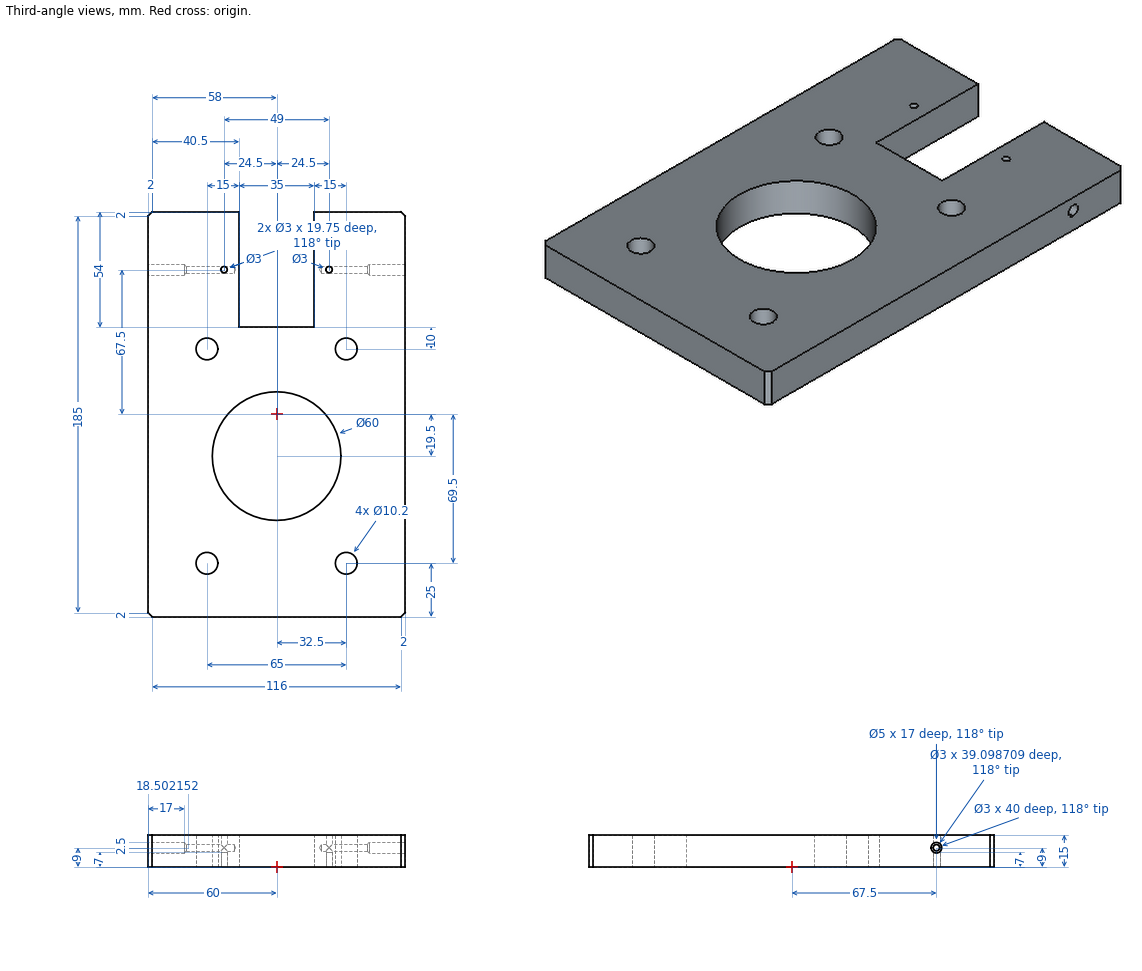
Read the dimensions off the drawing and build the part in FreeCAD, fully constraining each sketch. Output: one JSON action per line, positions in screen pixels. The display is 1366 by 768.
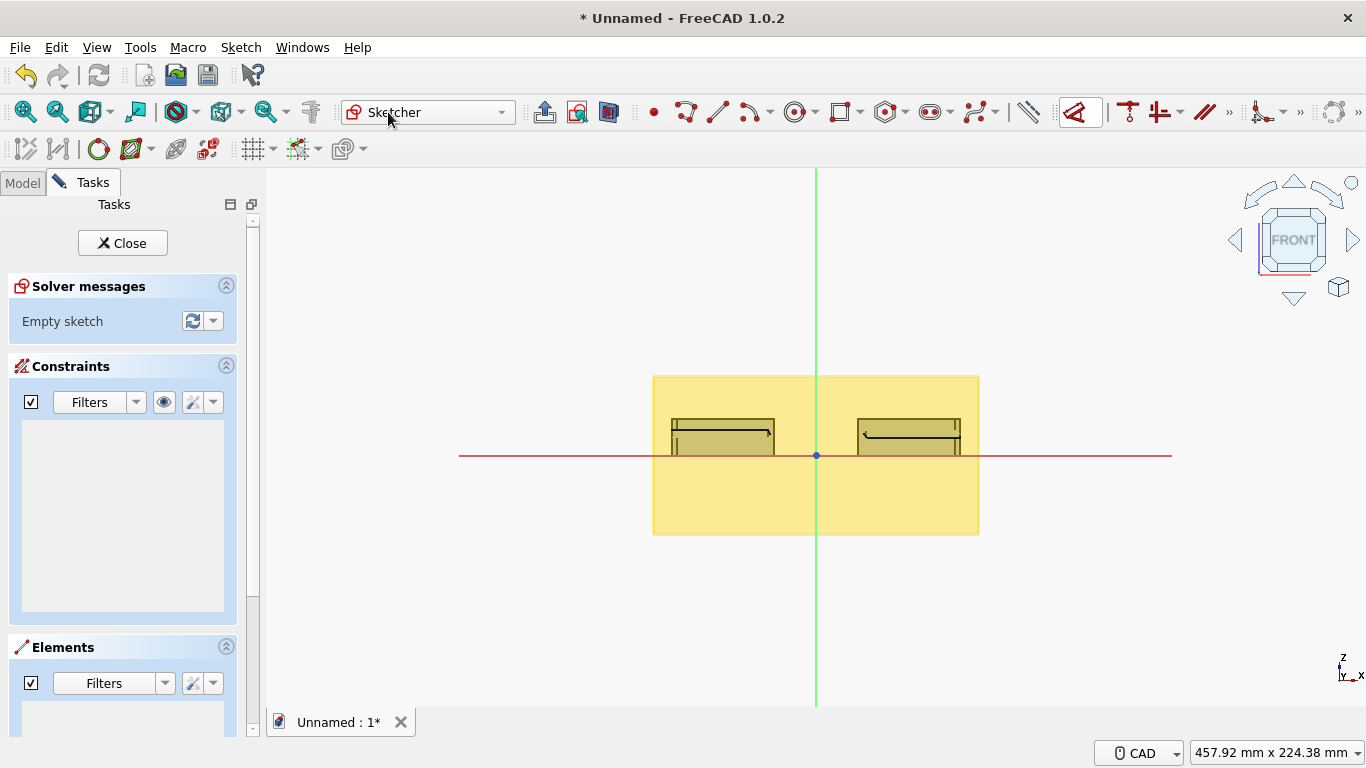
{"action": "scroll", "coordinate": [743, 443], "scroll_direction": "up", "scroll_amount": 7}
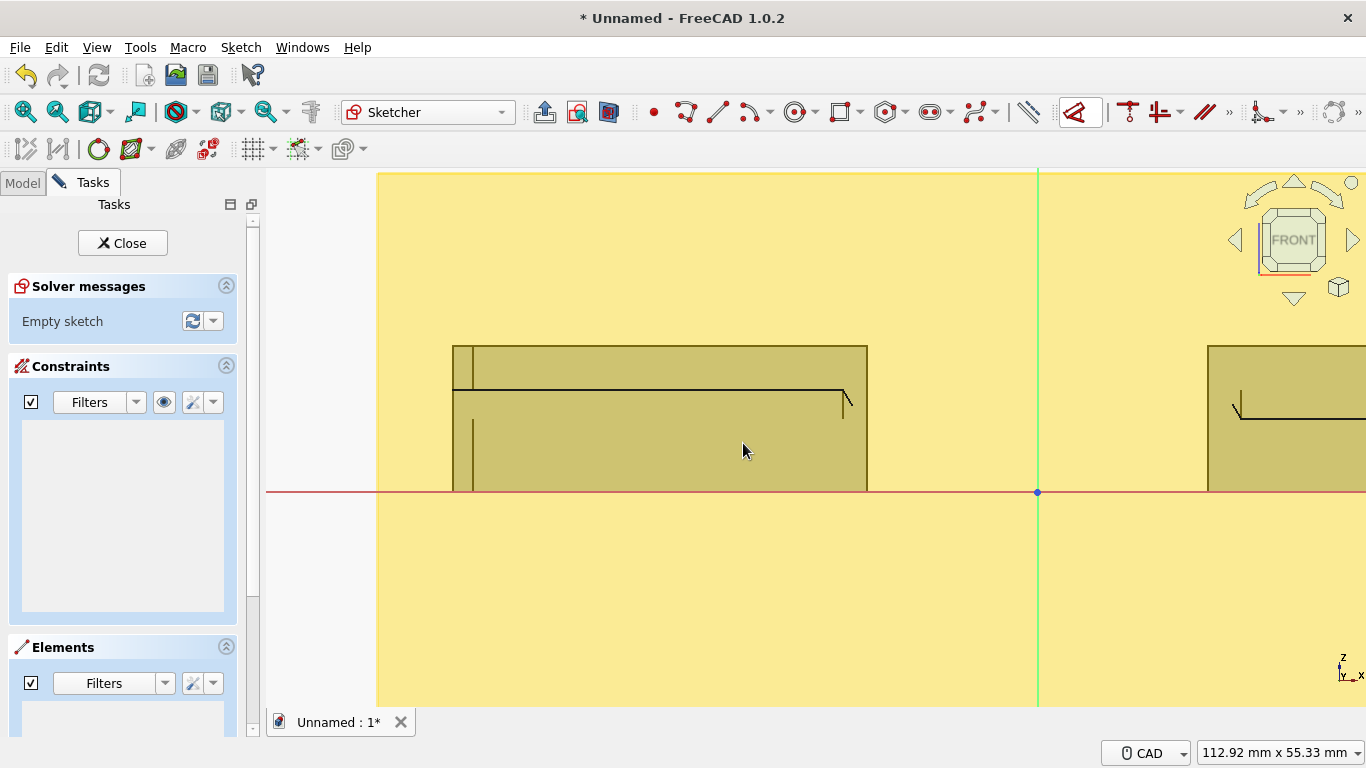
{"action": "left_click", "coordinate": [686, 112]}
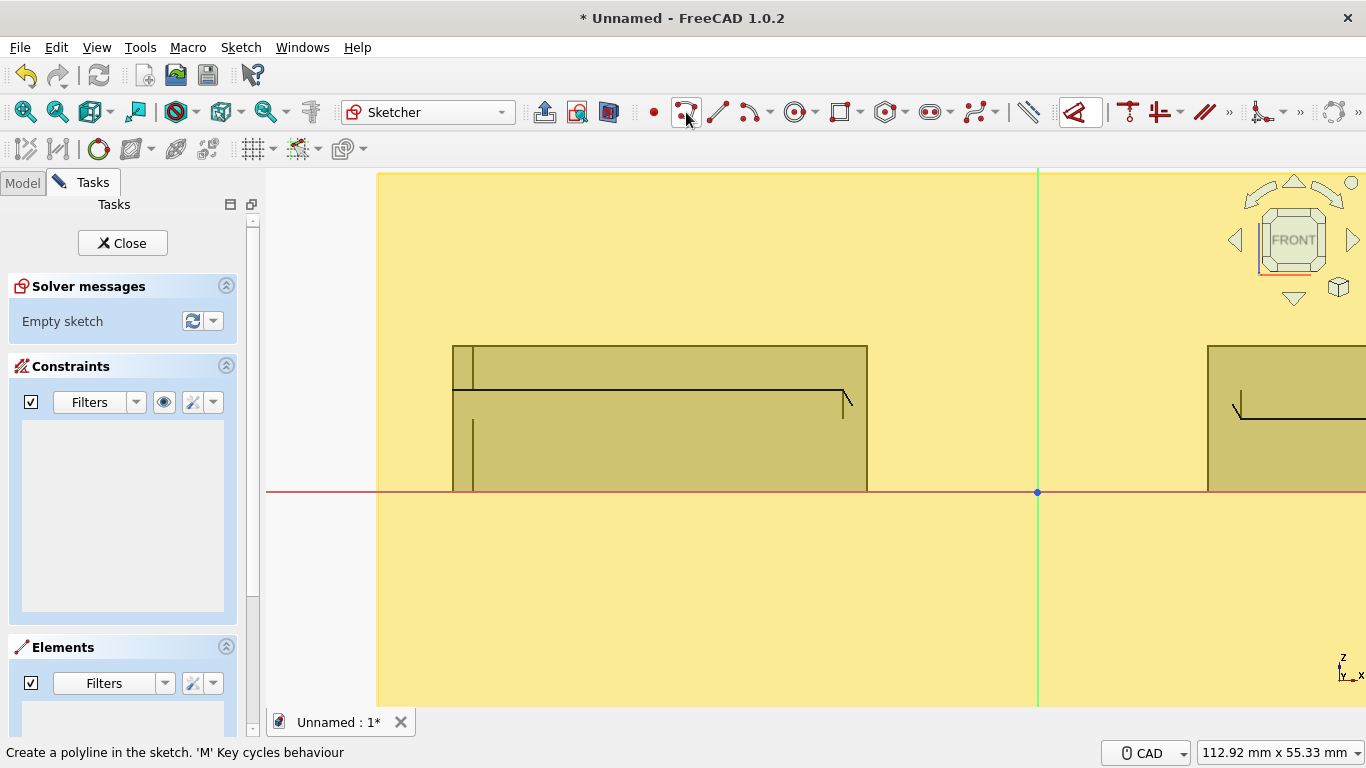
{"action": "left_click", "coordinate": [633, 405]}
{"action": "left_click", "coordinate": [453, 405]}
{"action": "left_click", "coordinate": [453, 380]}
{"action": "left_click", "coordinate": [619, 380]}
{"action": "left_click", "coordinate": [633, 406]}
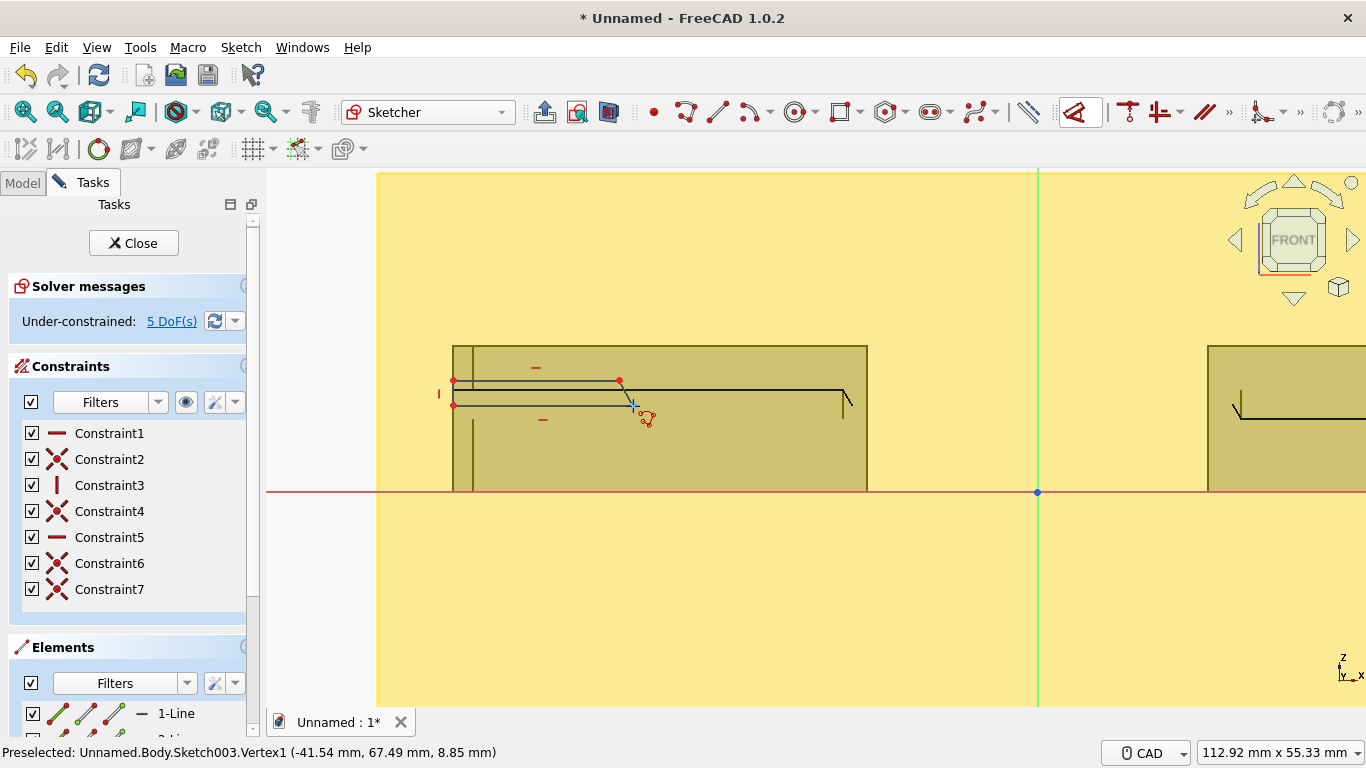
{"action": "left_click", "coordinate": [718, 112]}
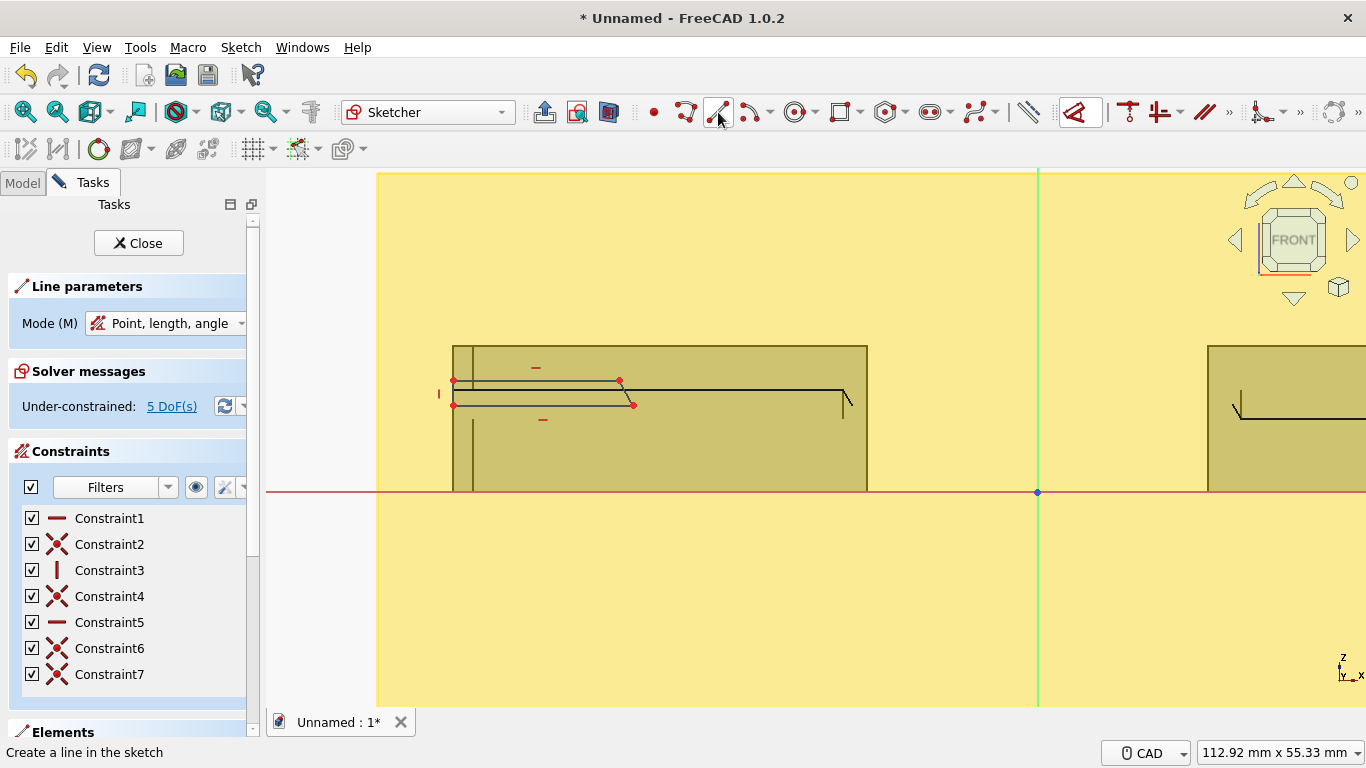
{"action": "left_click", "coordinate": [651, 405]}
{"action": "left_click", "coordinate": [706, 405]}
{"action": "key", "text": "Escape"}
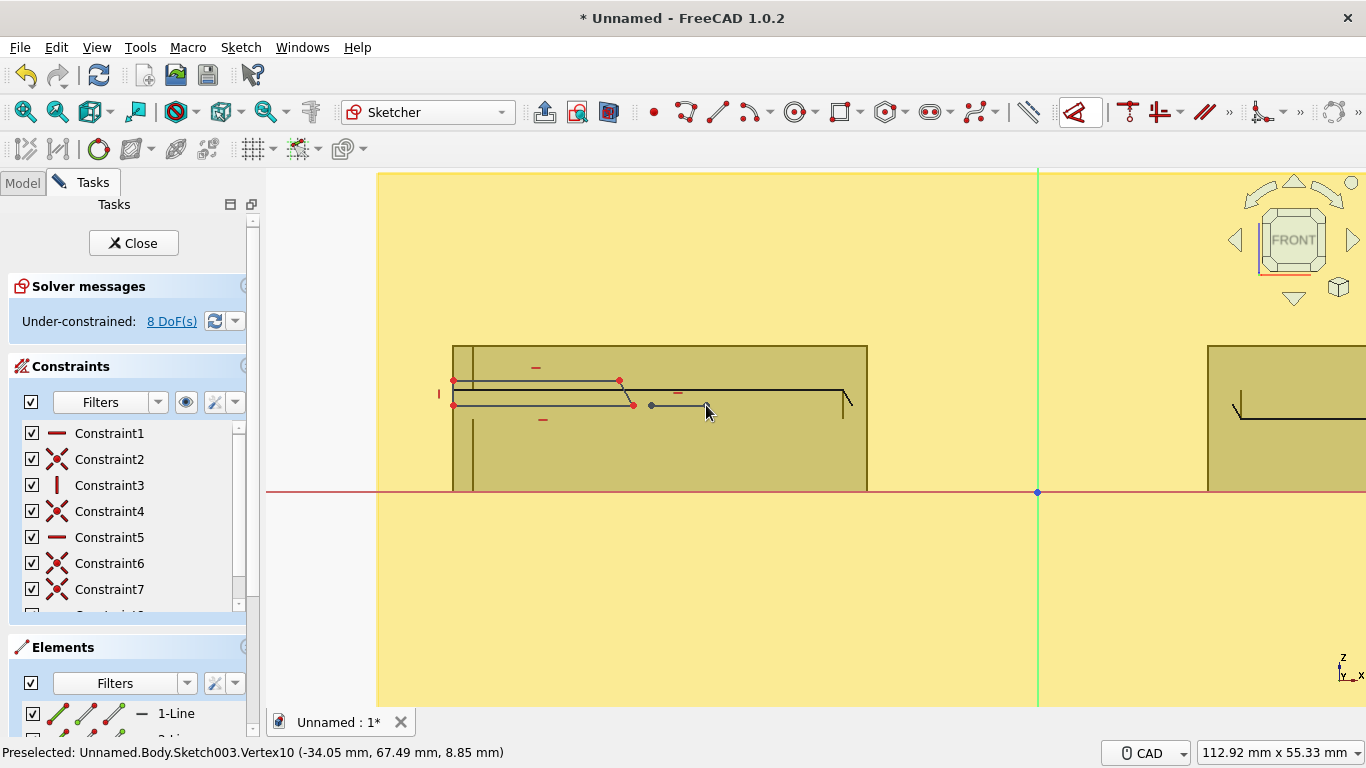
{"action": "left_click", "coordinate": [668, 406]}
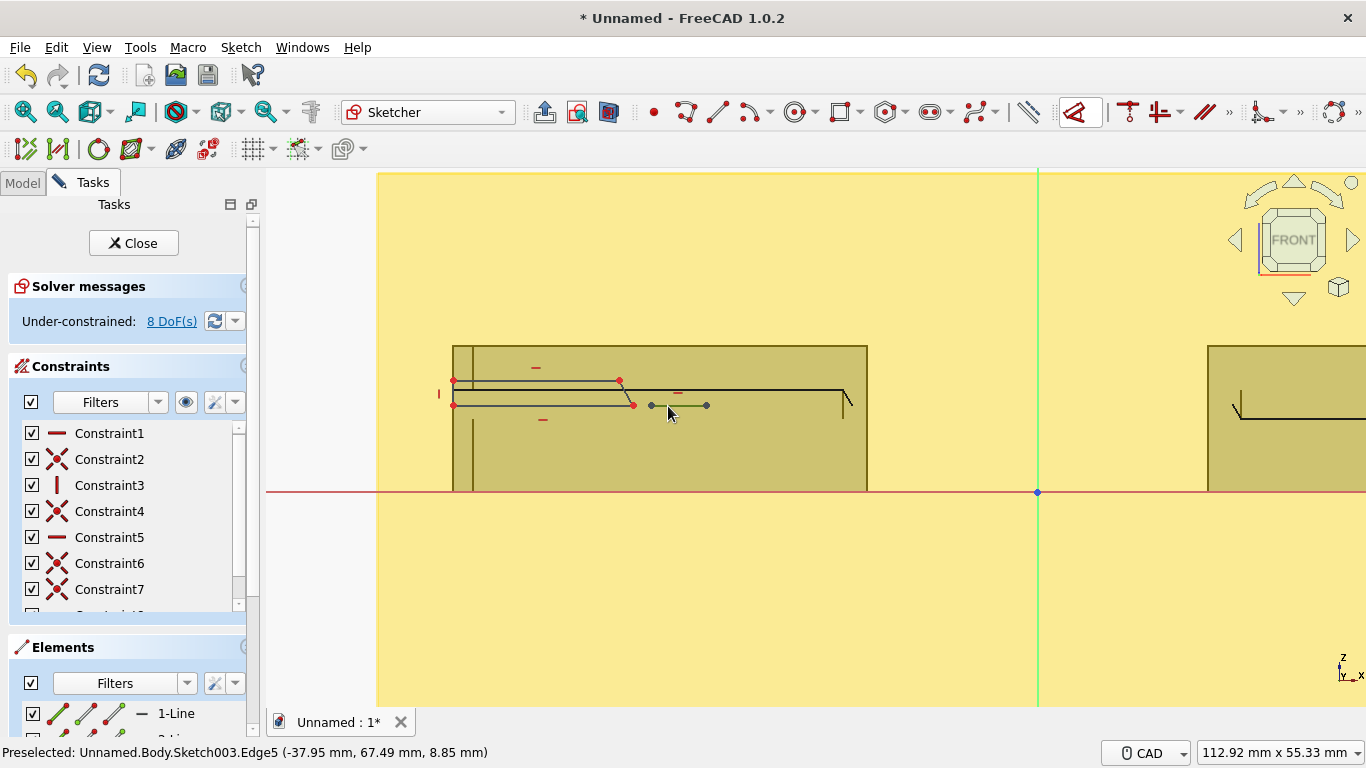
{"action": "left_click", "coordinate": [1030, 112]}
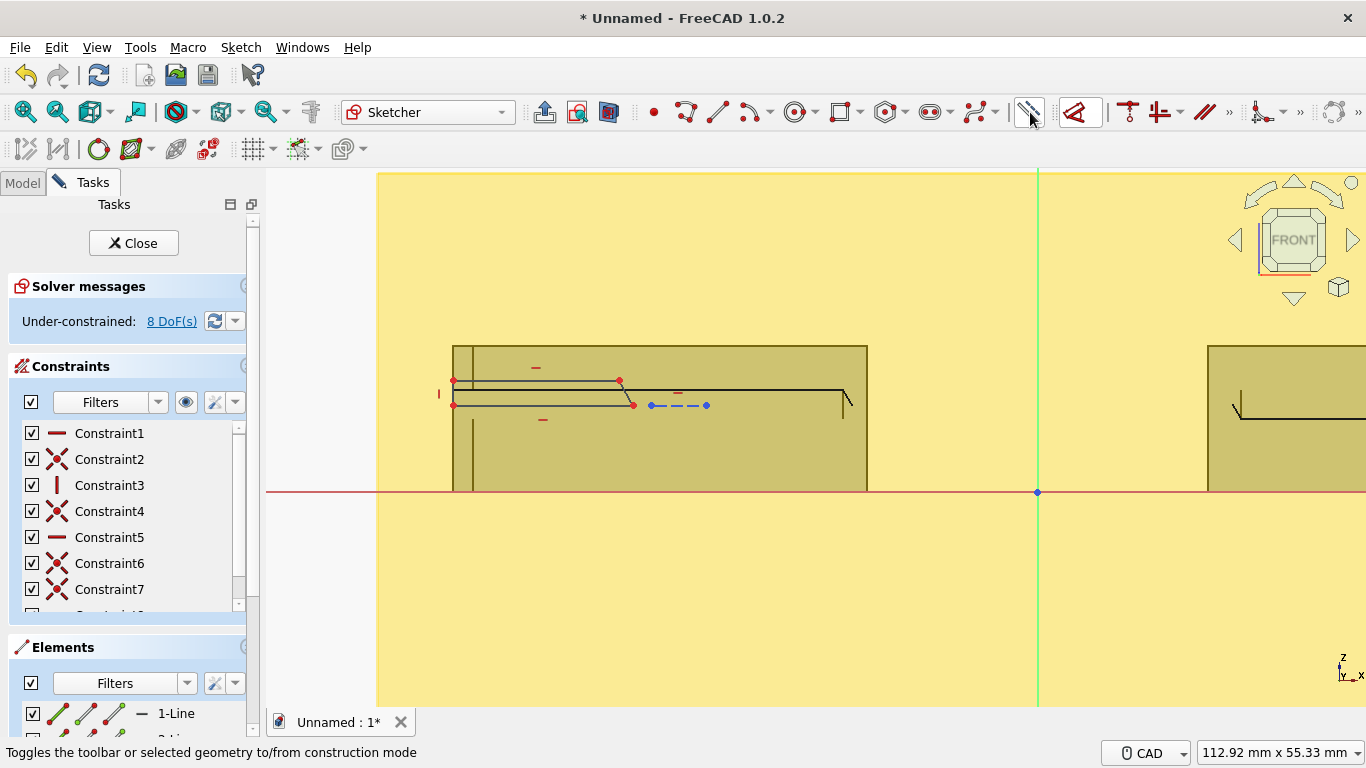
{"action": "left_click", "coordinate": [503, 381]}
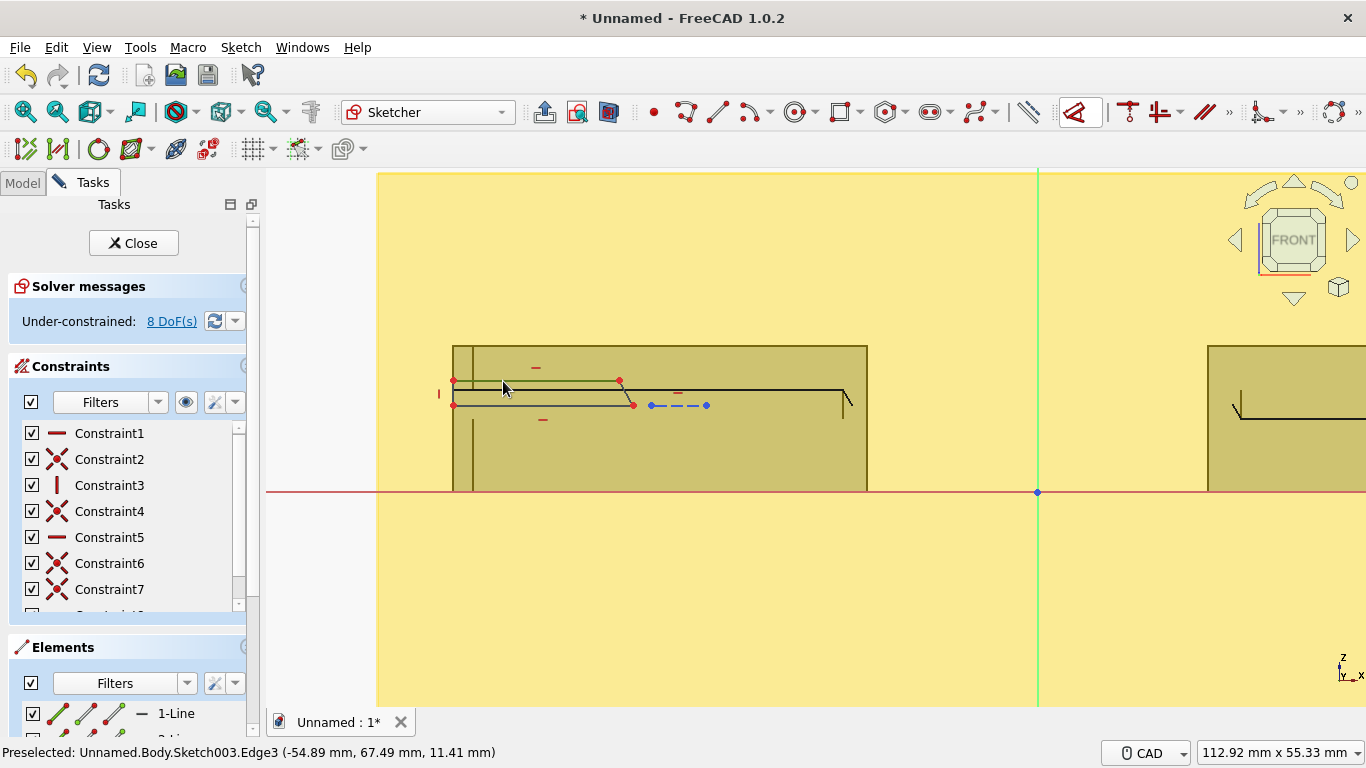
{"action": "key", "text": "l"}